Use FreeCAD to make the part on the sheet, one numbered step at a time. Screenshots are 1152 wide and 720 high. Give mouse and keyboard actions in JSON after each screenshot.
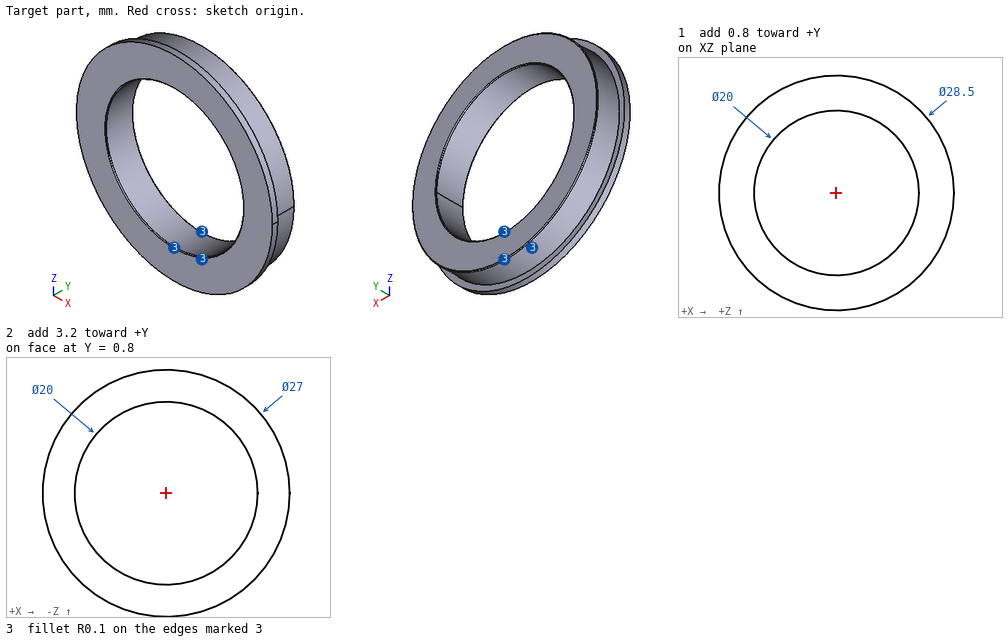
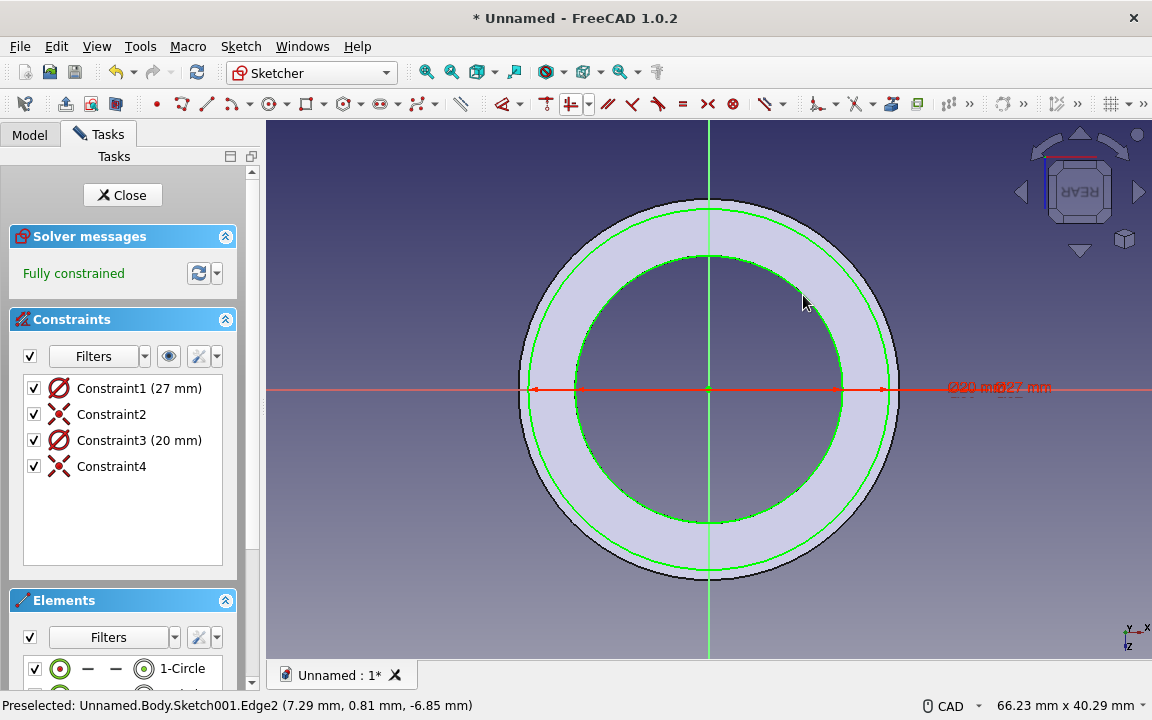
{"action": "left_click", "coordinate": [123, 195]}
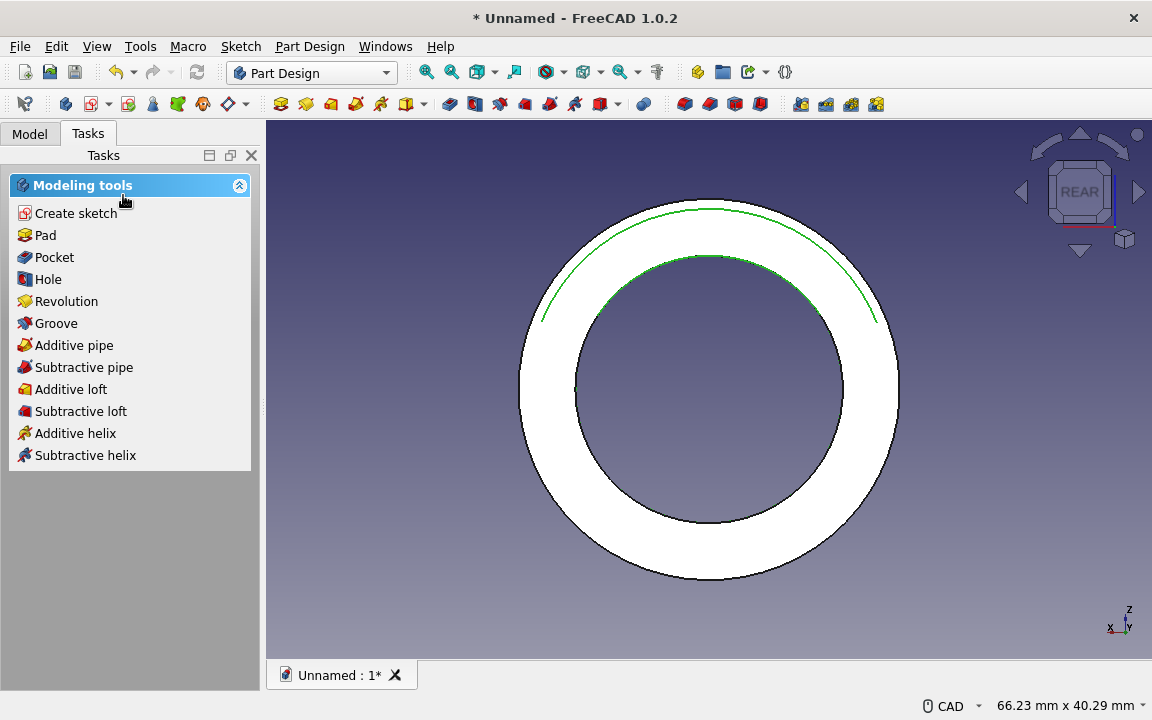
{"action": "left_click", "coordinate": [281, 104]}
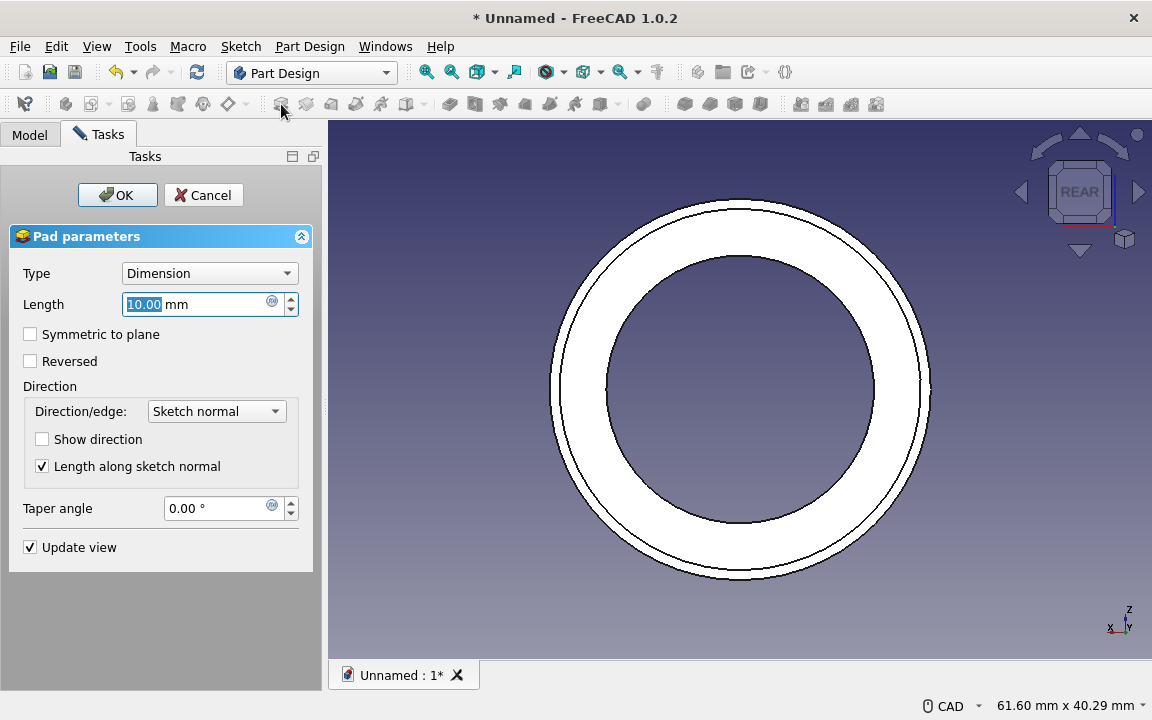
{"action": "type", "text": "3.2"}
{"action": "key", "text": "Tab"}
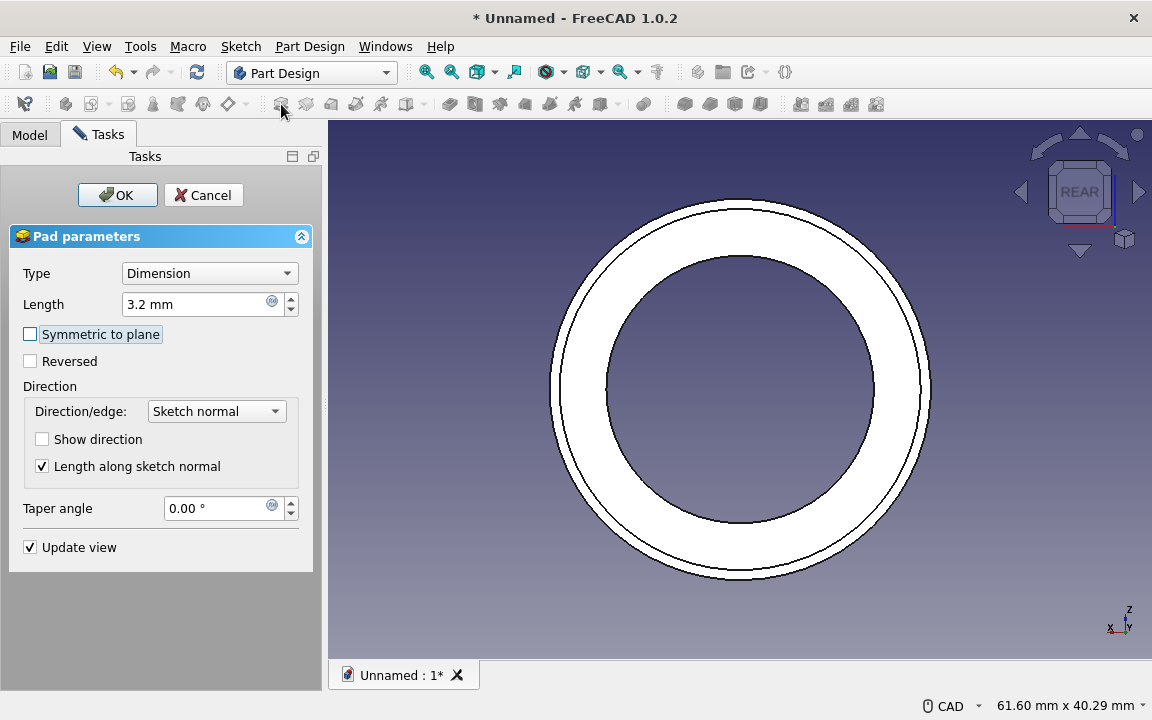
{"action": "left_click", "coordinate": [118, 195]}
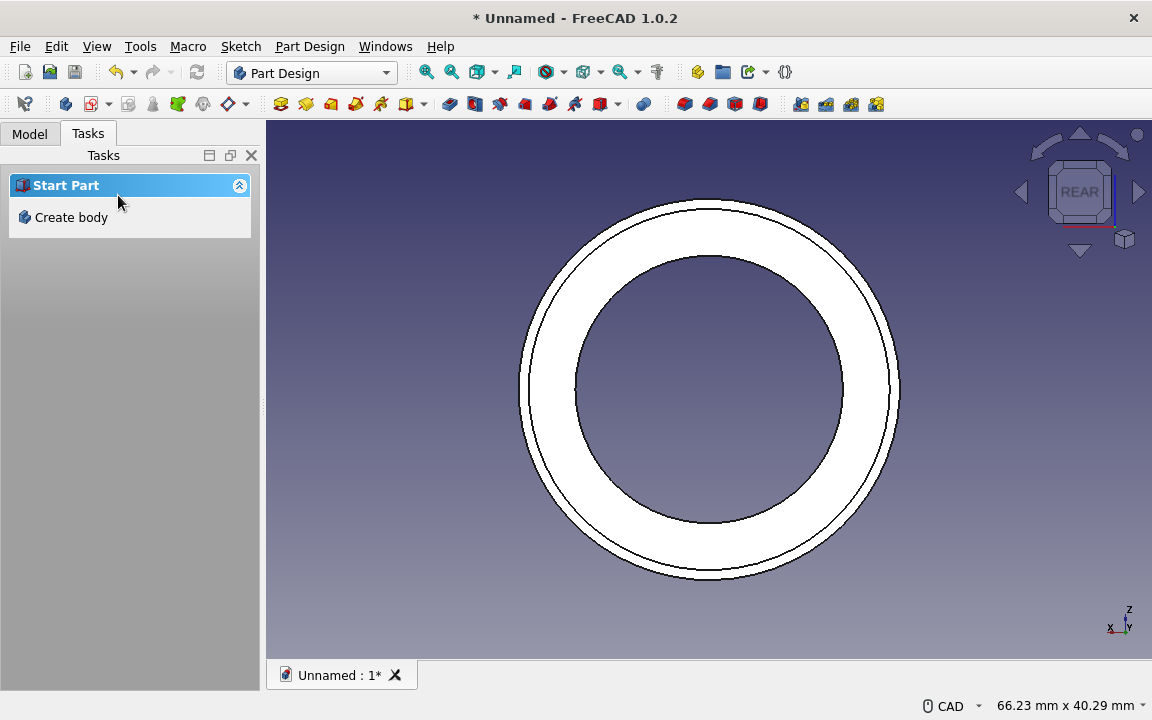
{"action": "left_click", "coordinate": [890, 389]}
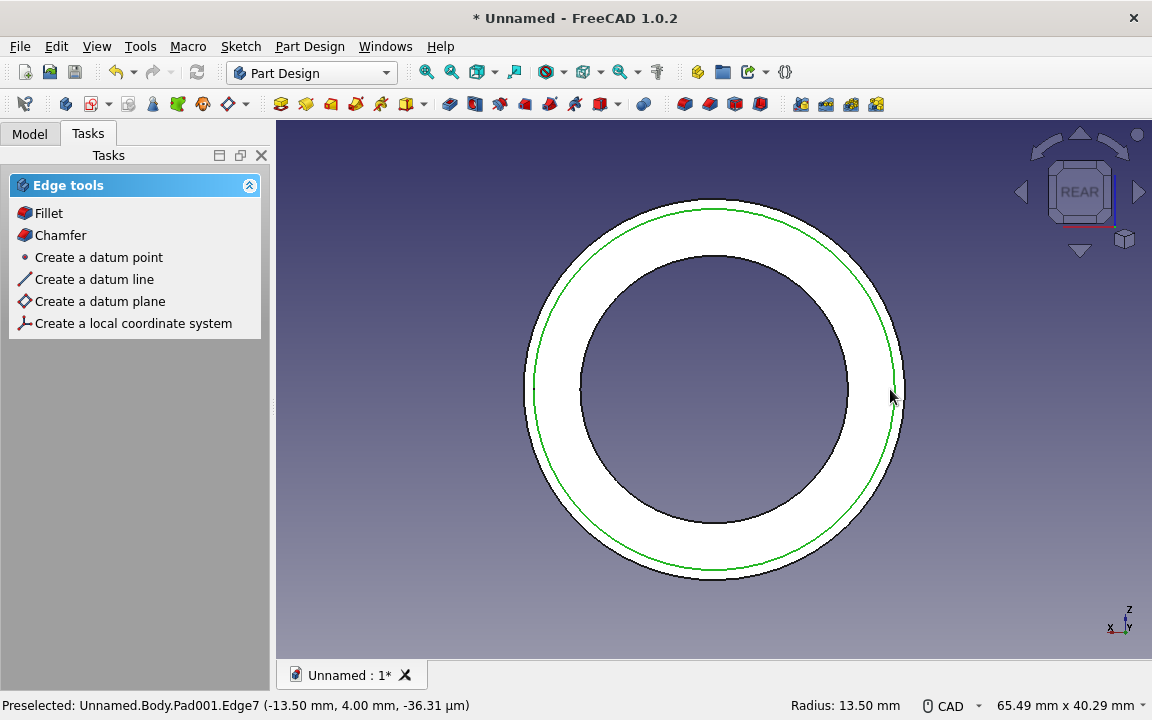
{"action": "left_click", "coordinate": [822, 310], "text": "ctrl"}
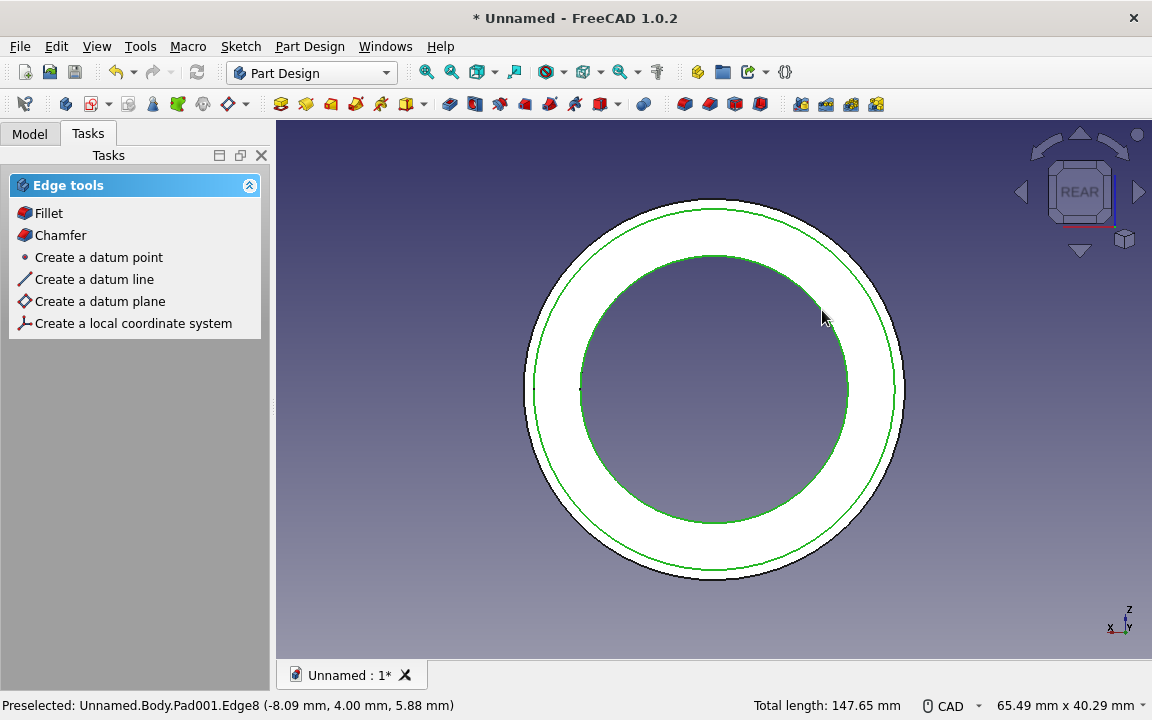
{"action": "key", "text": "0"}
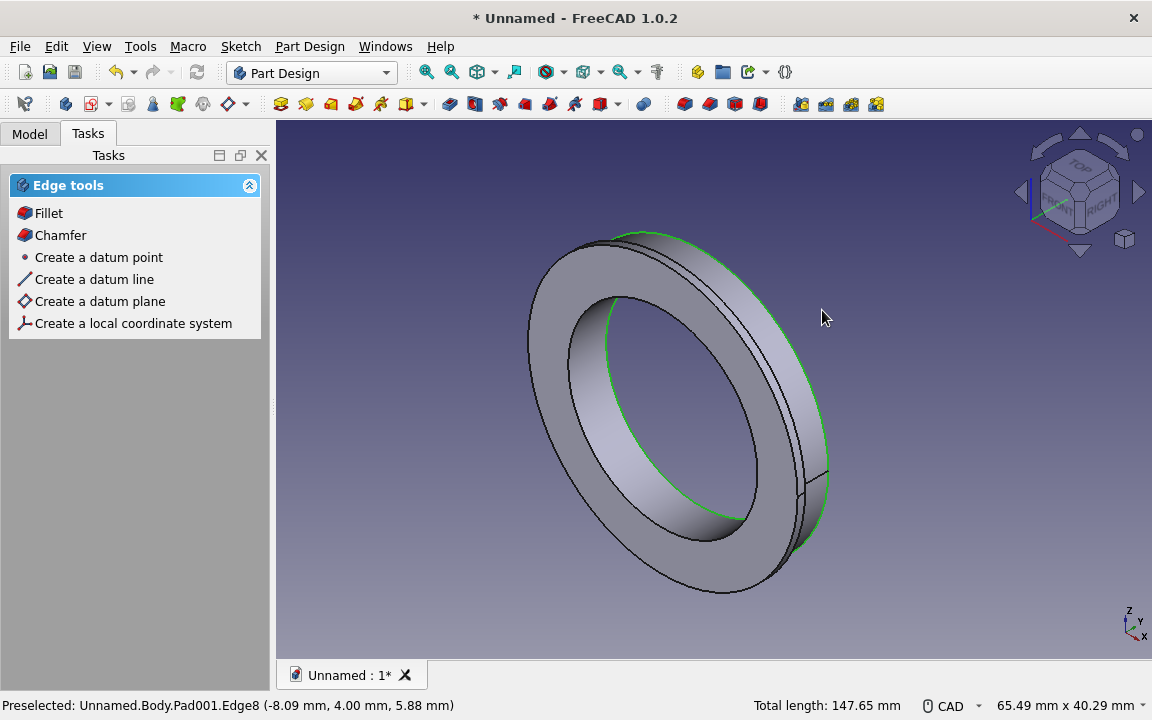
{"action": "left_click", "coordinate": [568, 363], "text": "ctrl"}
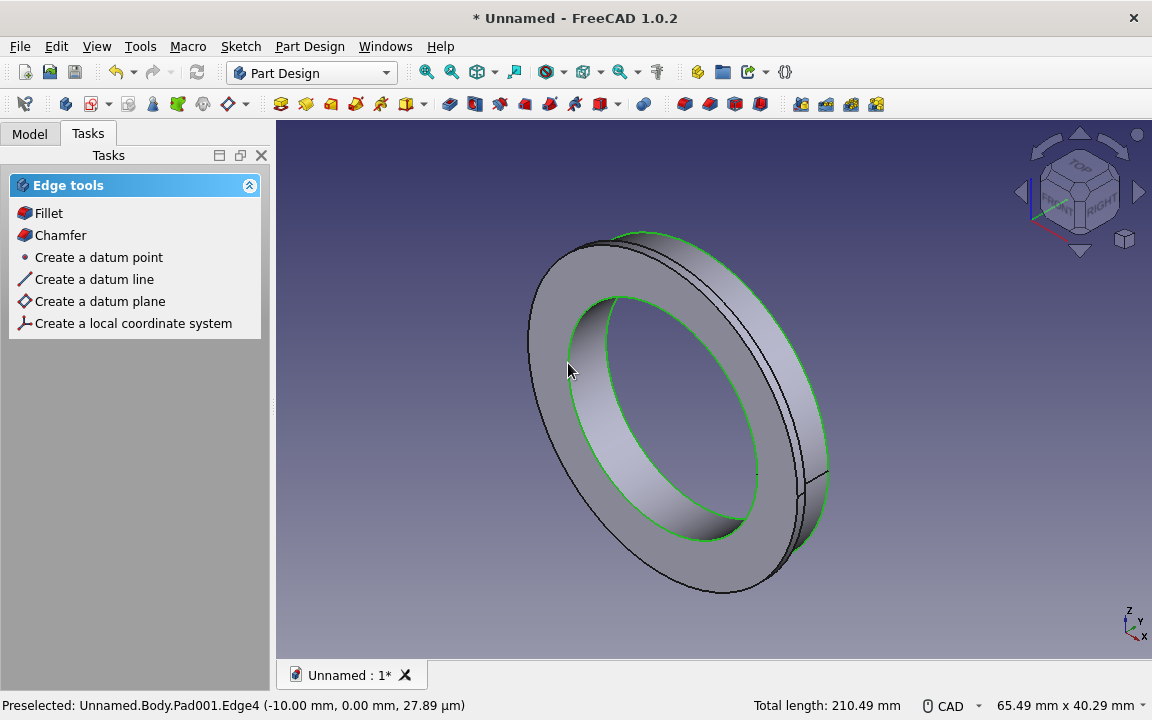
{"action": "left_click", "coordinate": [685, 104]}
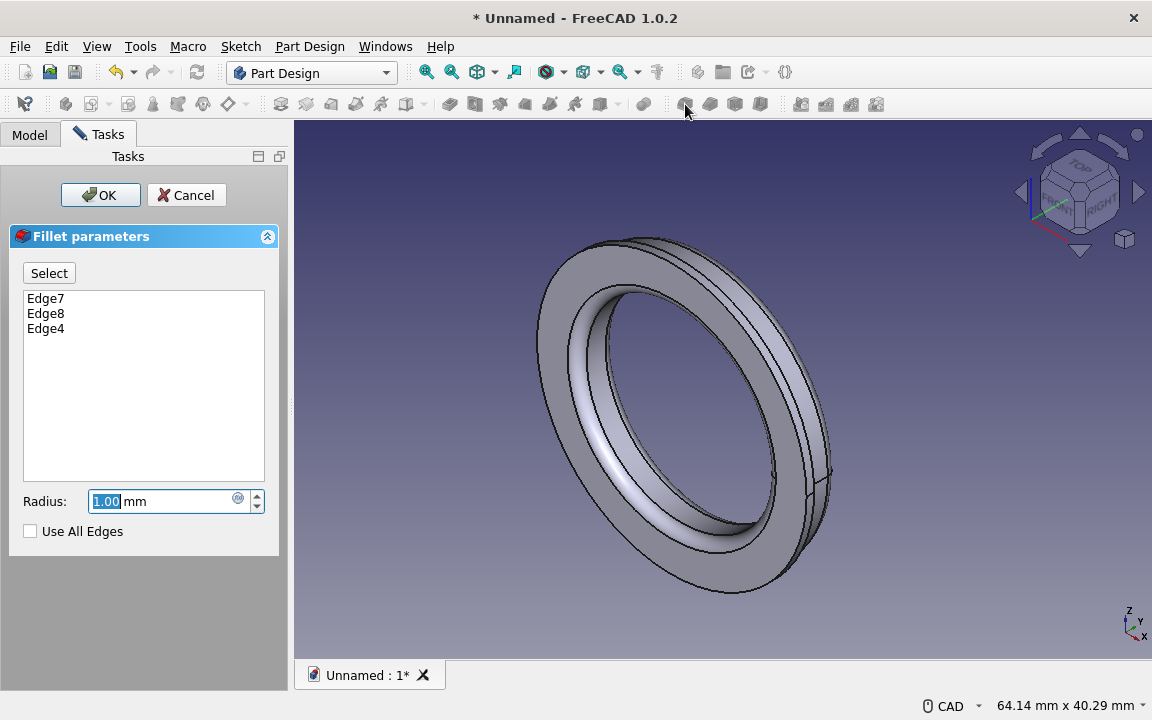
{"action": "type", "text": "0.1"}
{"action": "key", "text": "Tab"}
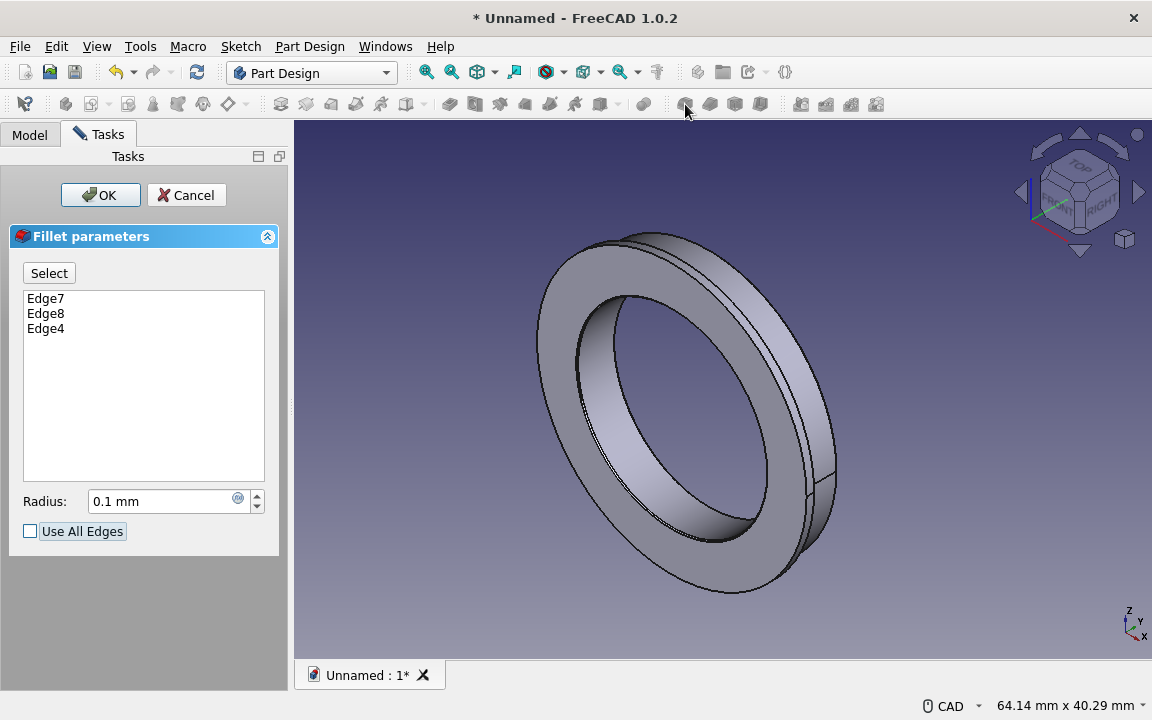
{"action": "left_click", "coordinate": [101, 195]}